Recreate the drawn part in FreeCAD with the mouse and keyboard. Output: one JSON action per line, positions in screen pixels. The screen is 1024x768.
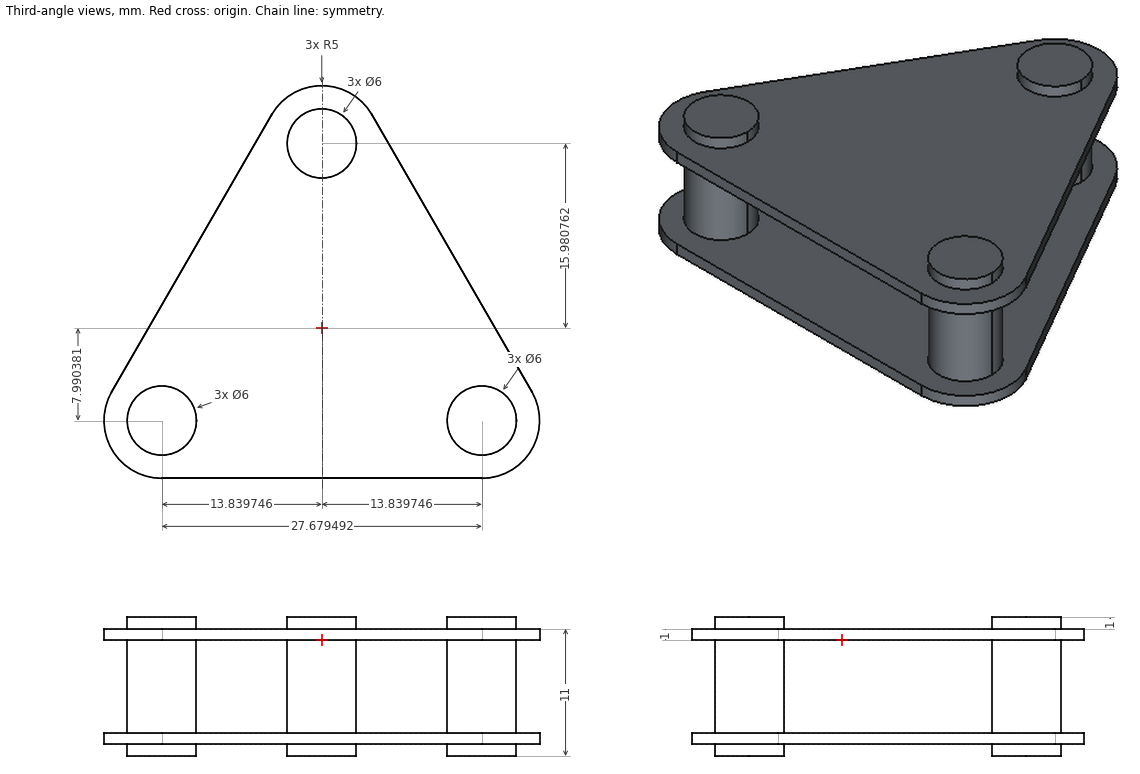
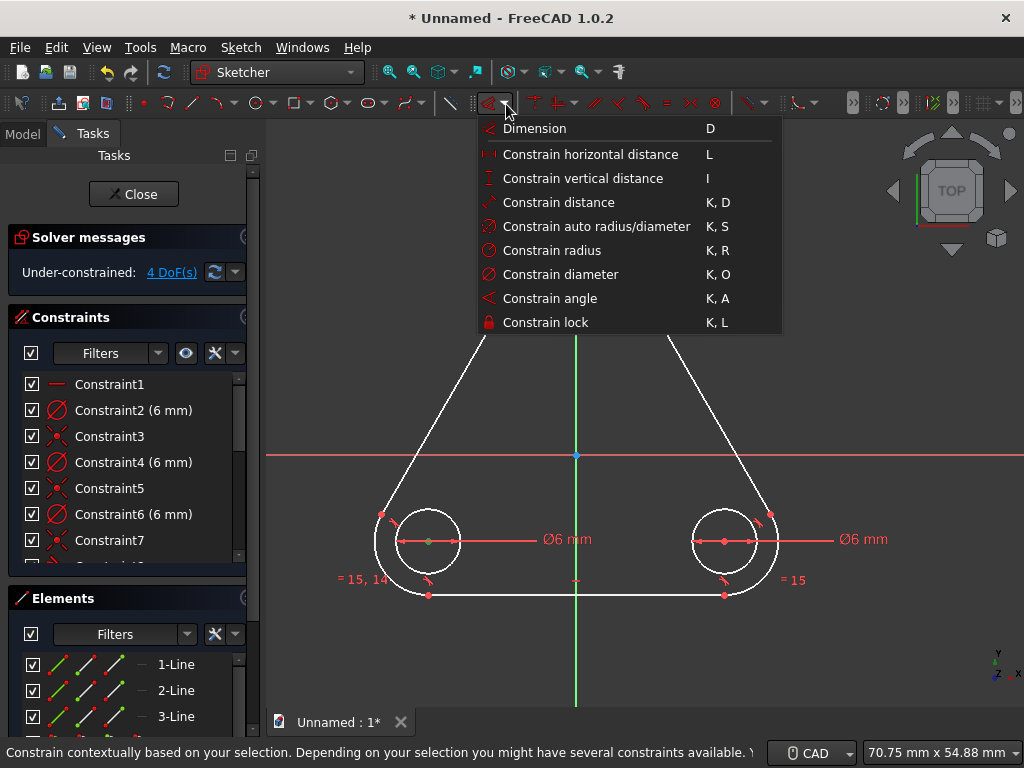
{"action": "left_click", "coordinate": [630, 178]}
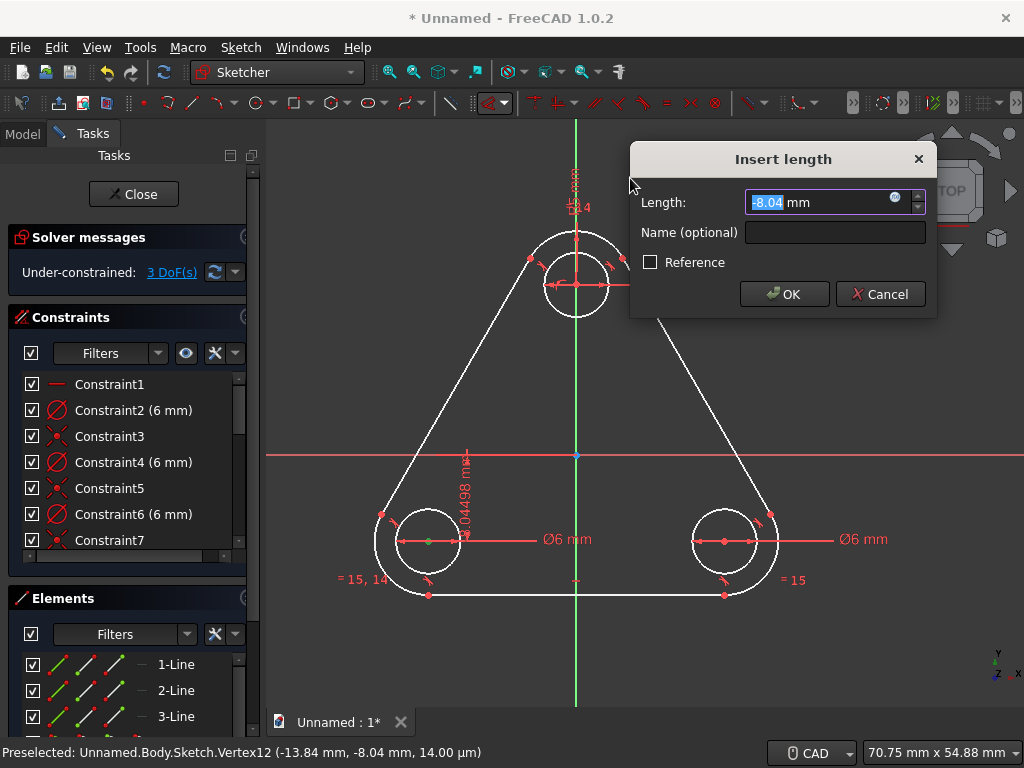
{"action": "type", "text": "-7.990381"}
{"action": "key", "text": "Return"}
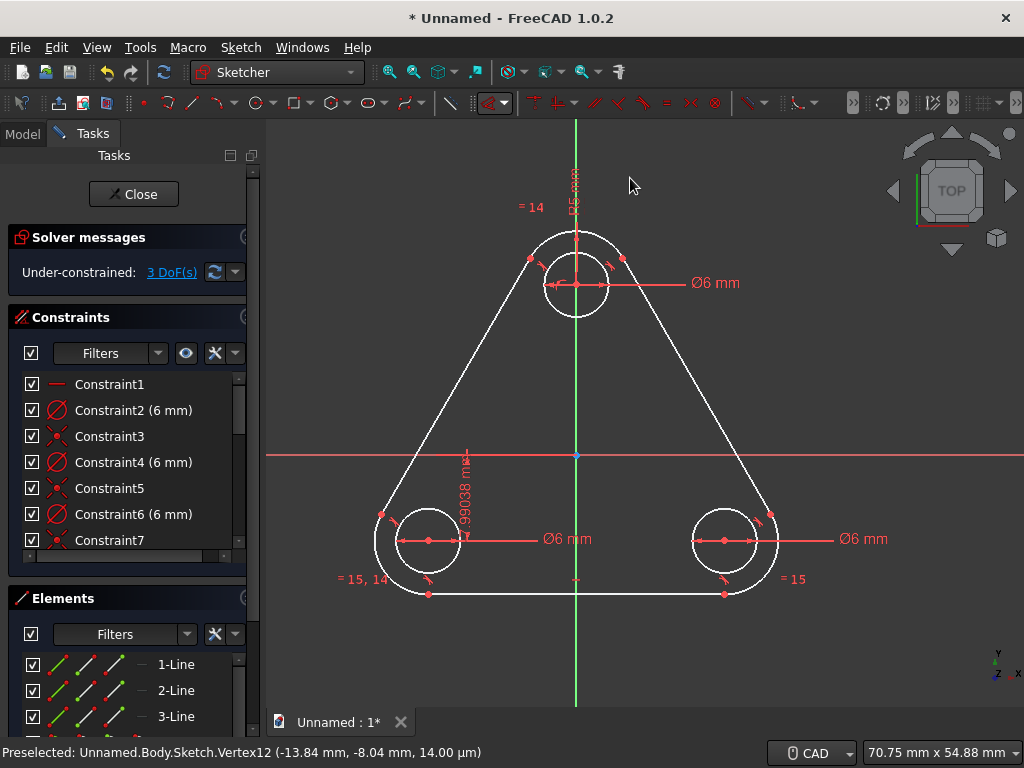
{"action": "left_click", "coordinate": [517, 594]}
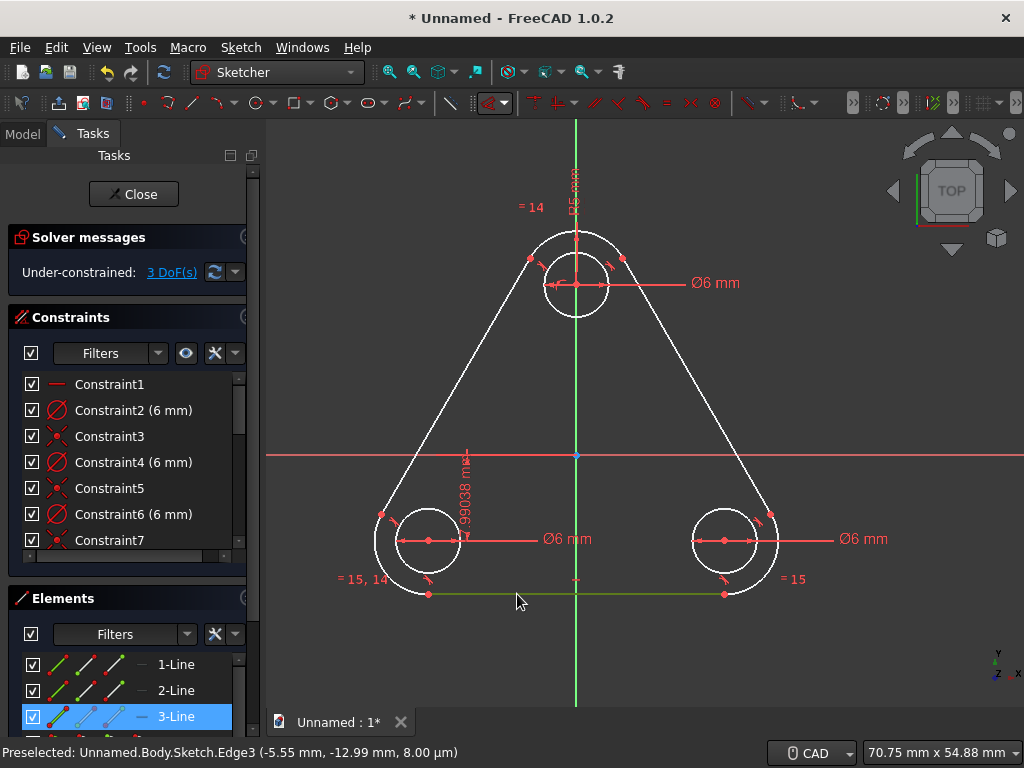
{"action": "left_click", "coordinate": [506, 104]}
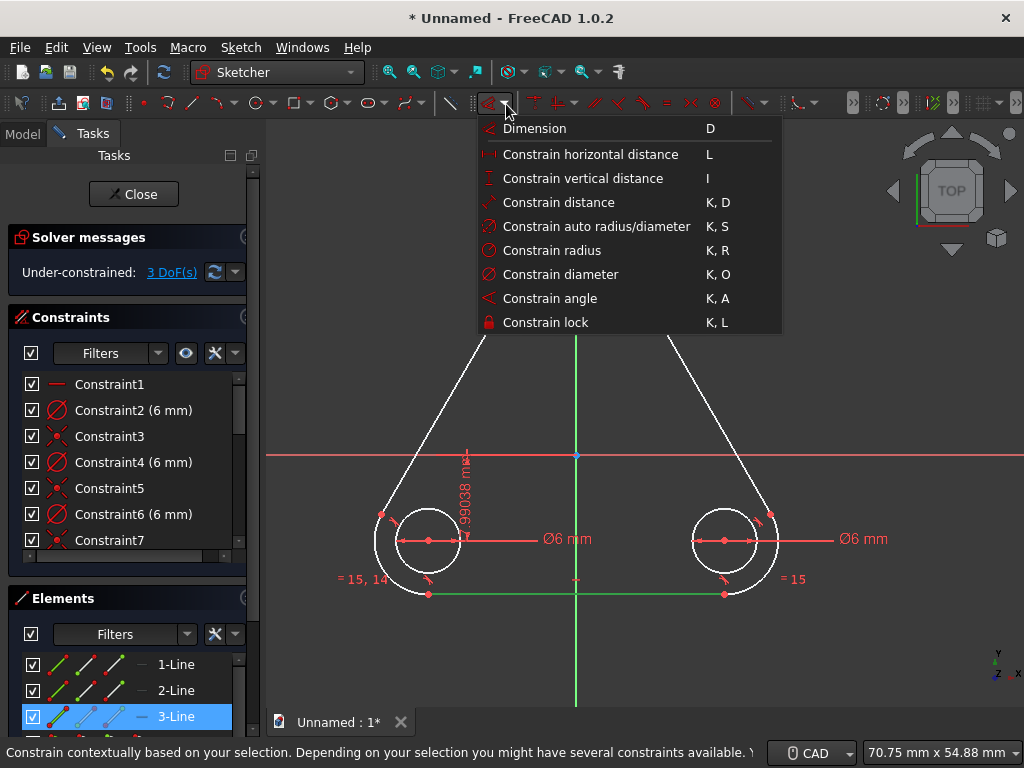
{"action": "left_click", "coordinate": [630, 154]}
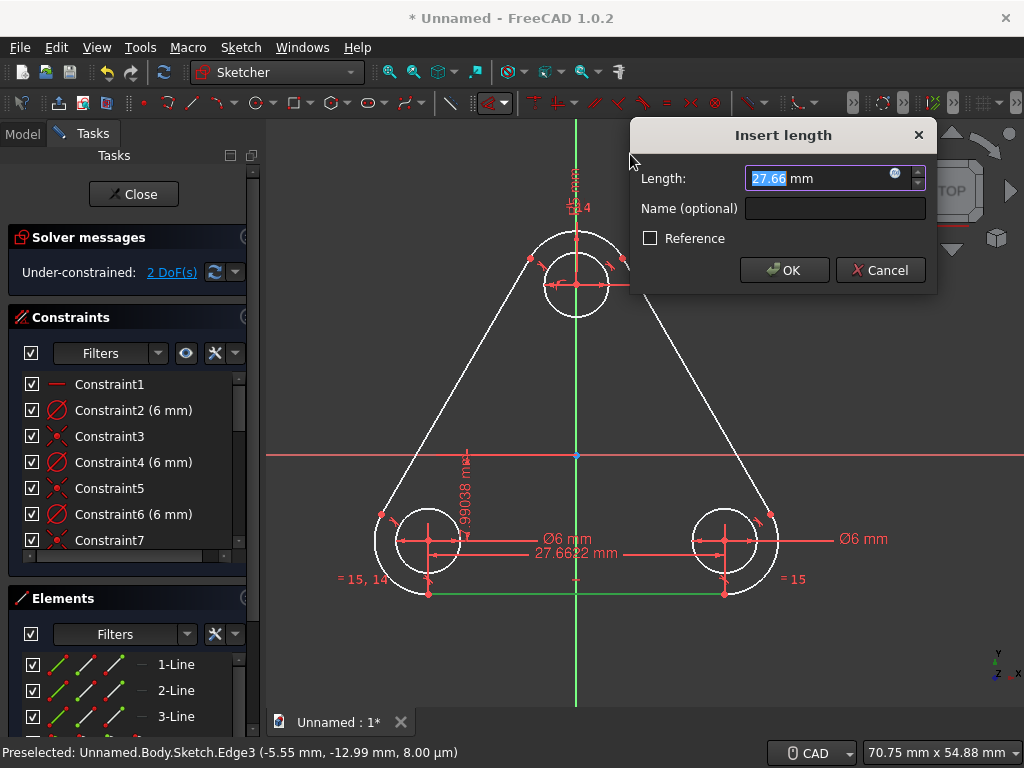
{"action": "type", "text": "27.679492"}
{"action": "key", "text": "Return"}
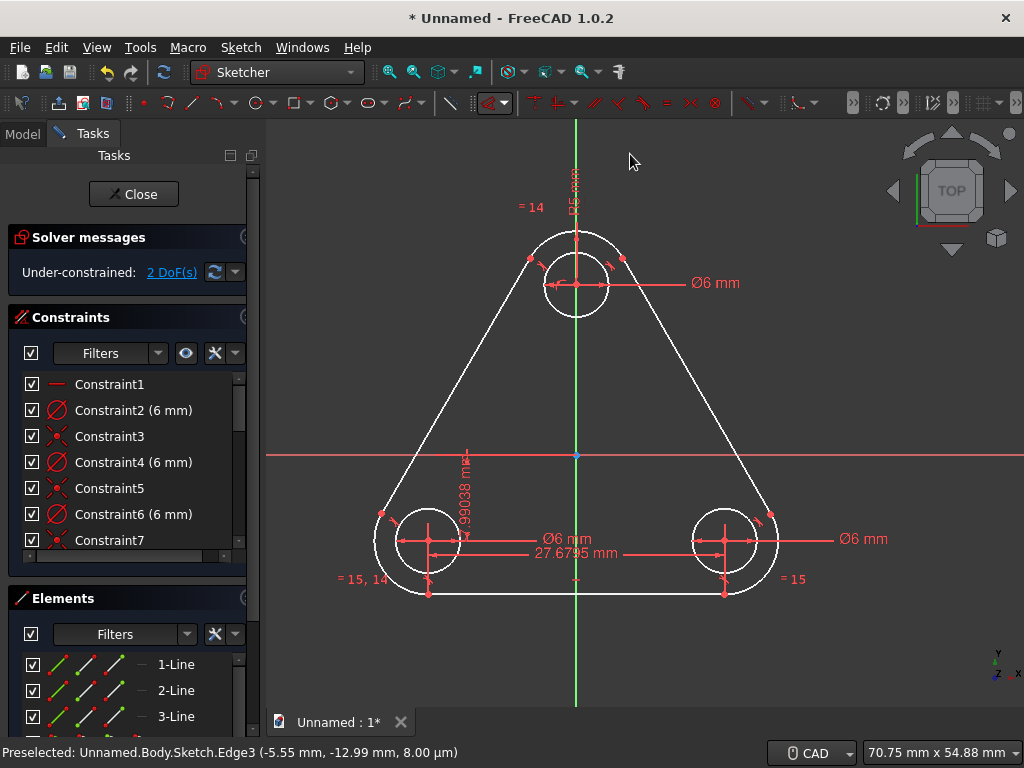
{"action": "left_click", "coordinate": [428, 541]}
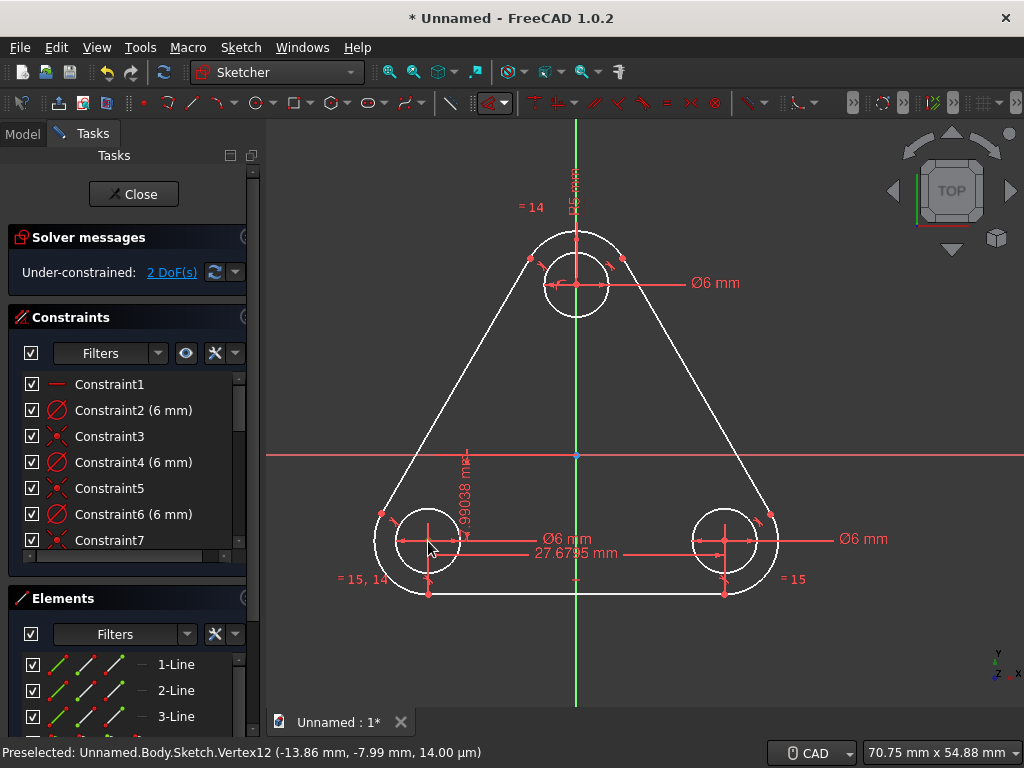
{"action": "key", "text": "l"}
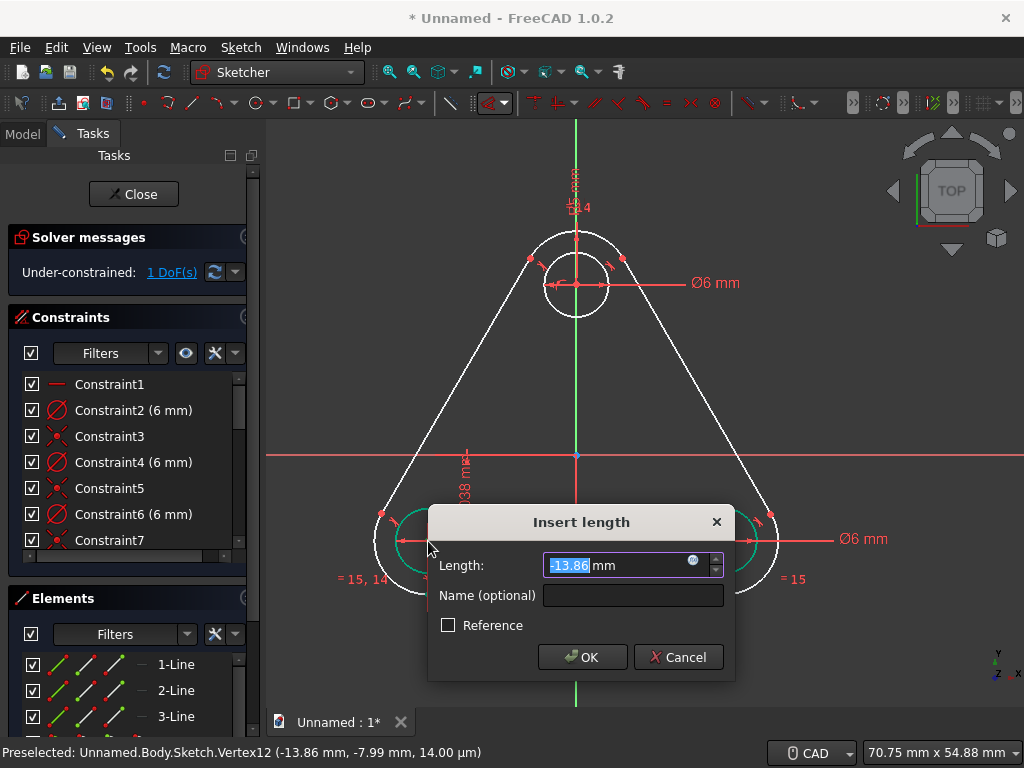
{"action": "type", "text": "-13.839746"}
{"action": "key", "text": "Return"}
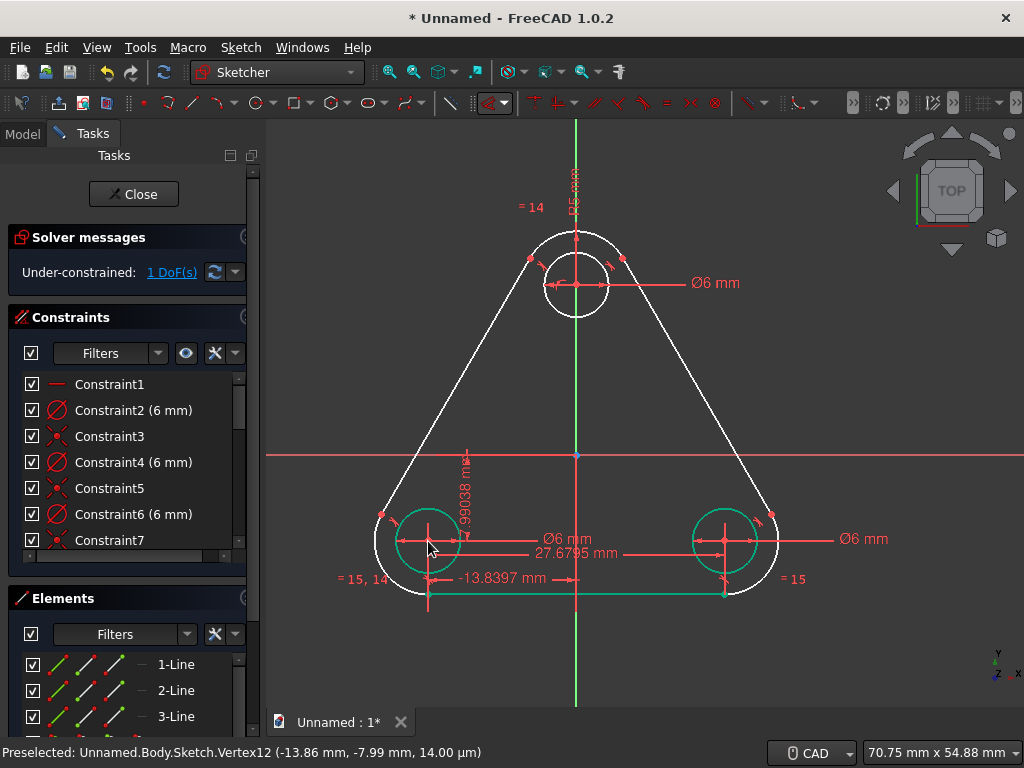
{"action": "left_click", "coordinate": [576, 285]}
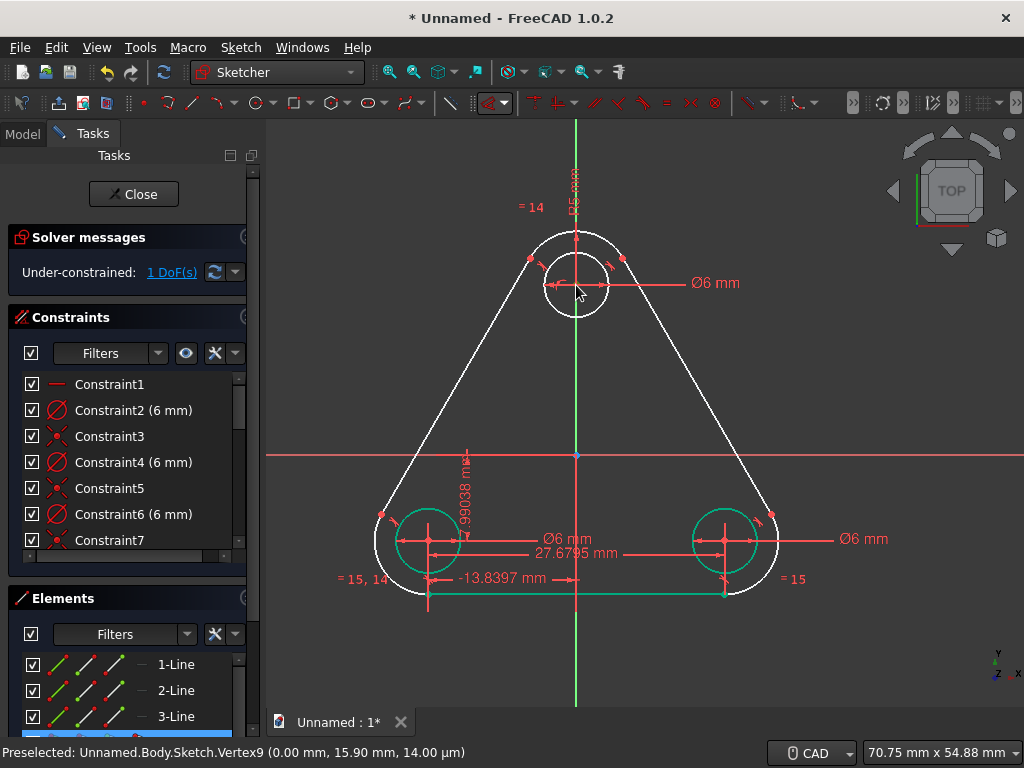
{"action": "key", "text": "i"}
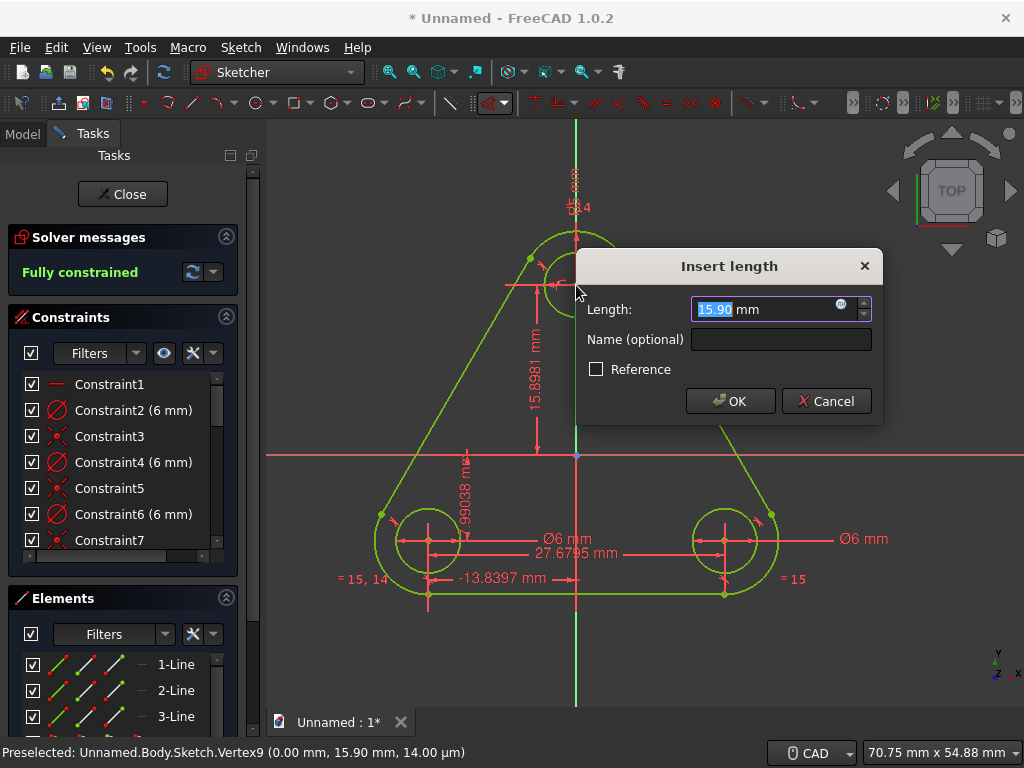
{"action": "type", "text": "15.980762"}
{"action": "key", "text": "Return"}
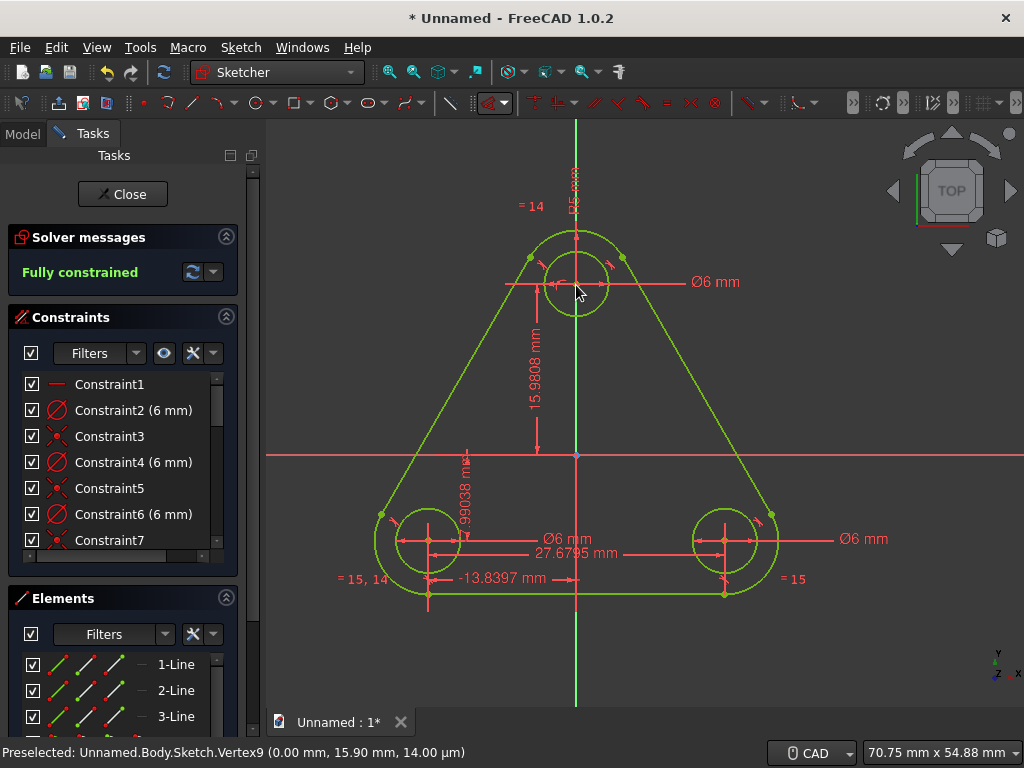
{"action": "left_click", "coordinate": [123, 194]}